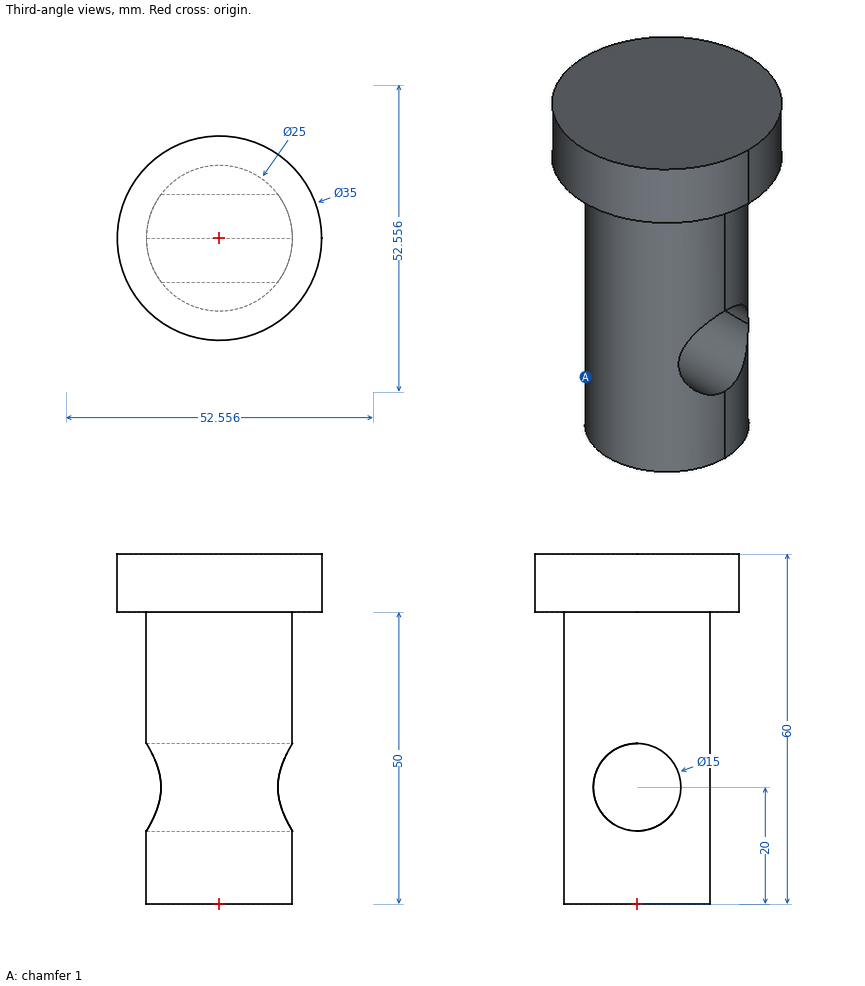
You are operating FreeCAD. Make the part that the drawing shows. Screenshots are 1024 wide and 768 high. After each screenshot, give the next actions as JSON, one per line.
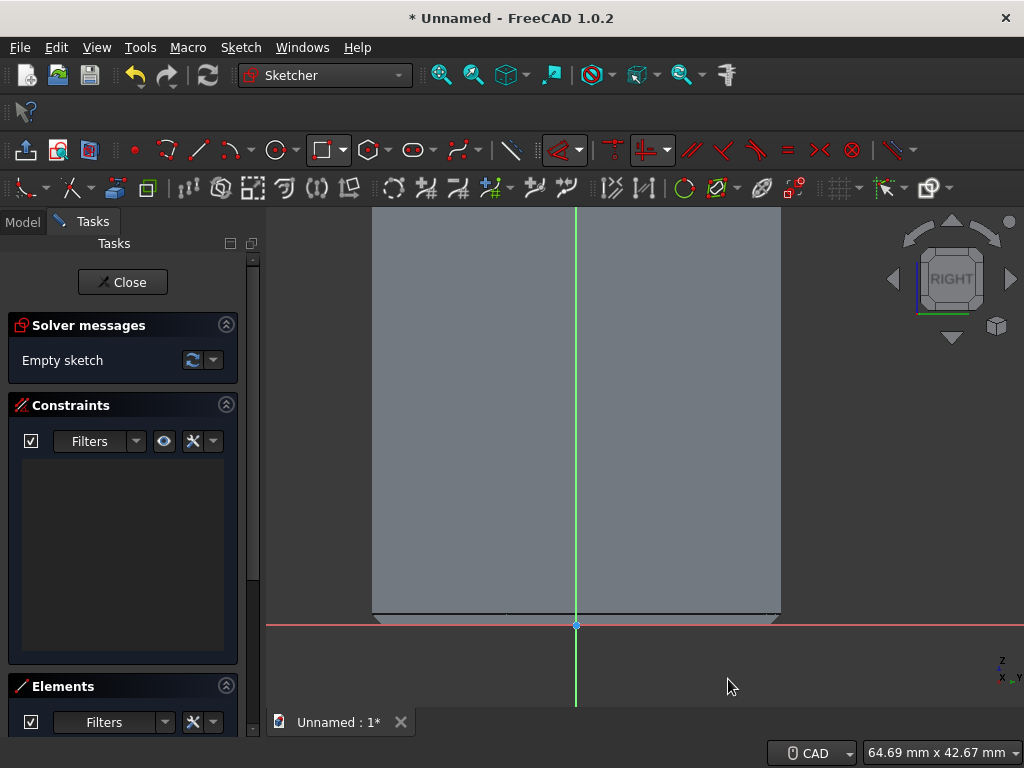
{"action": "left_click", "coordinate": [276, 150]}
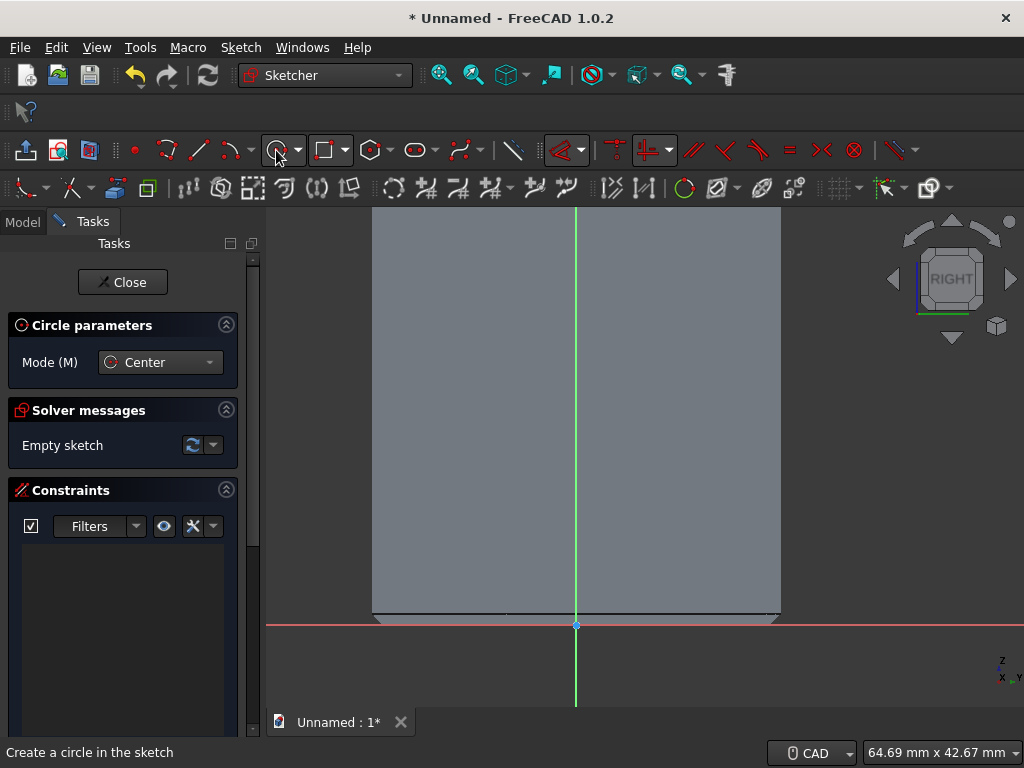
{"action": "left_click", "coordinate": [576, 391]}
{"action": "left_click", "coordinate": [638, 329]}
{"action": "key", "text": "Escape"}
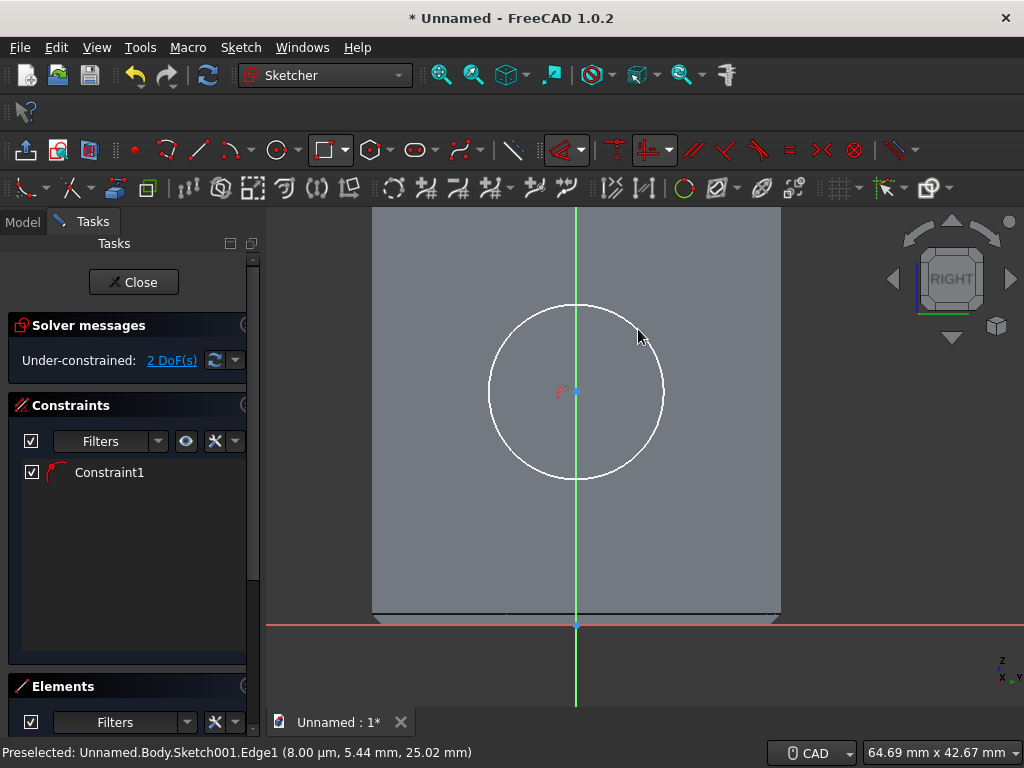
{"action": "left_click", "coordinate": [638, 330]}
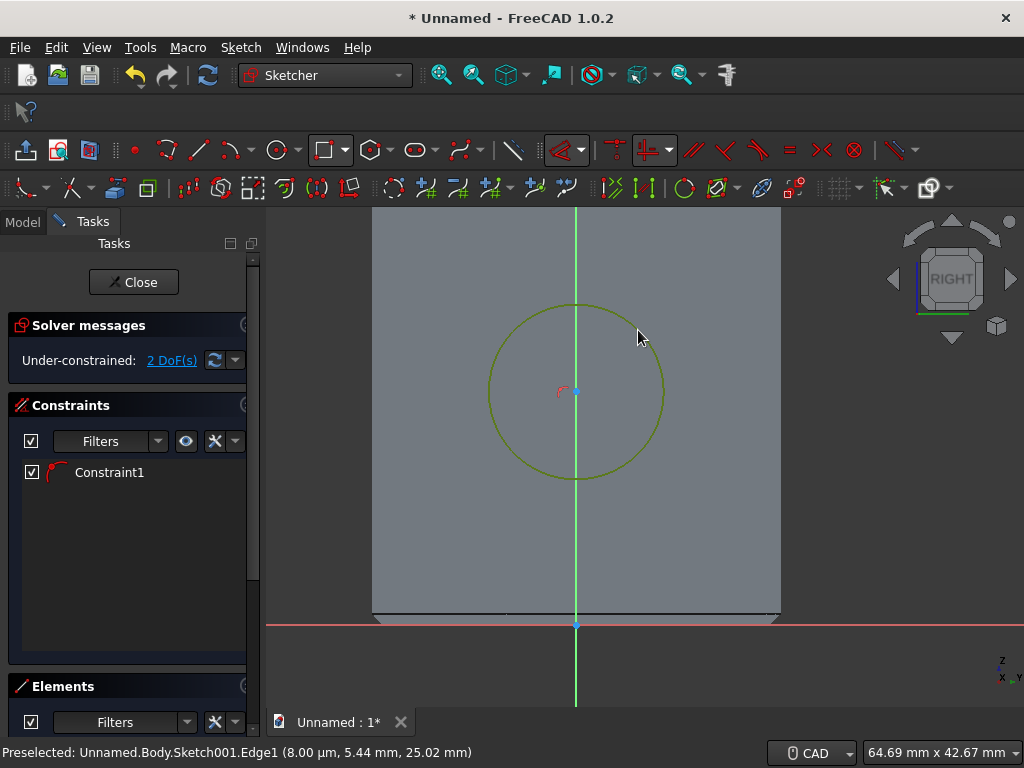
{"action": "key", "text": "k o"}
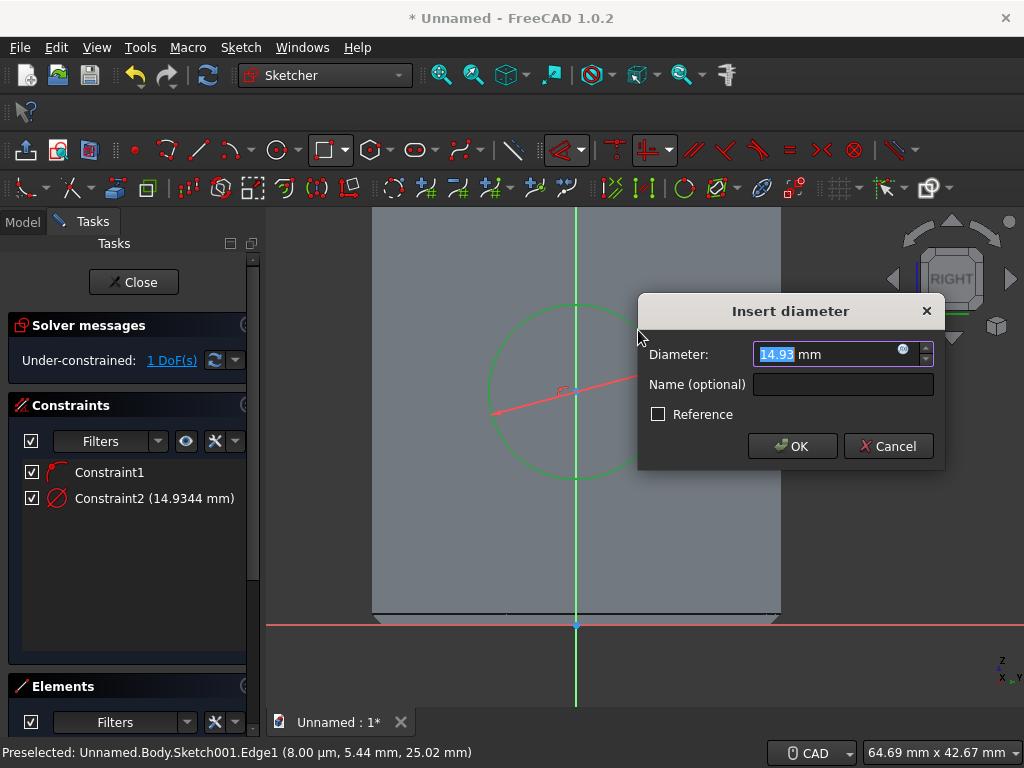
{"action": "type", "text": "15"}
{"action": "key", "text": "Return"}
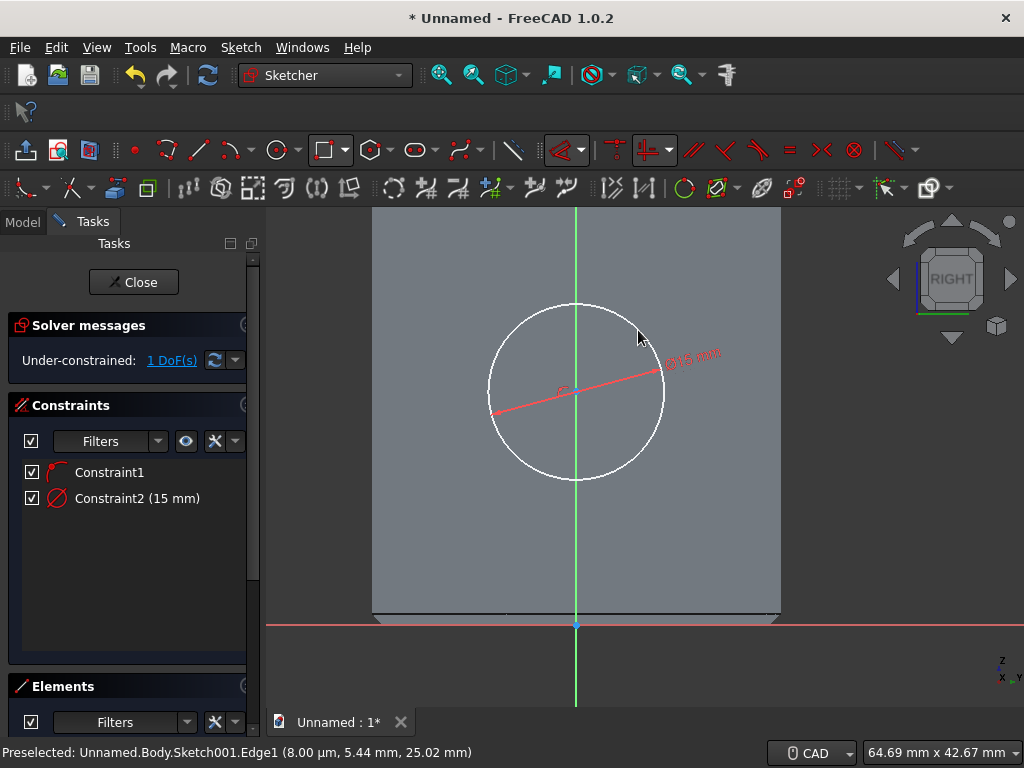
{"action": "left_click", "coordinate": [576, 392]}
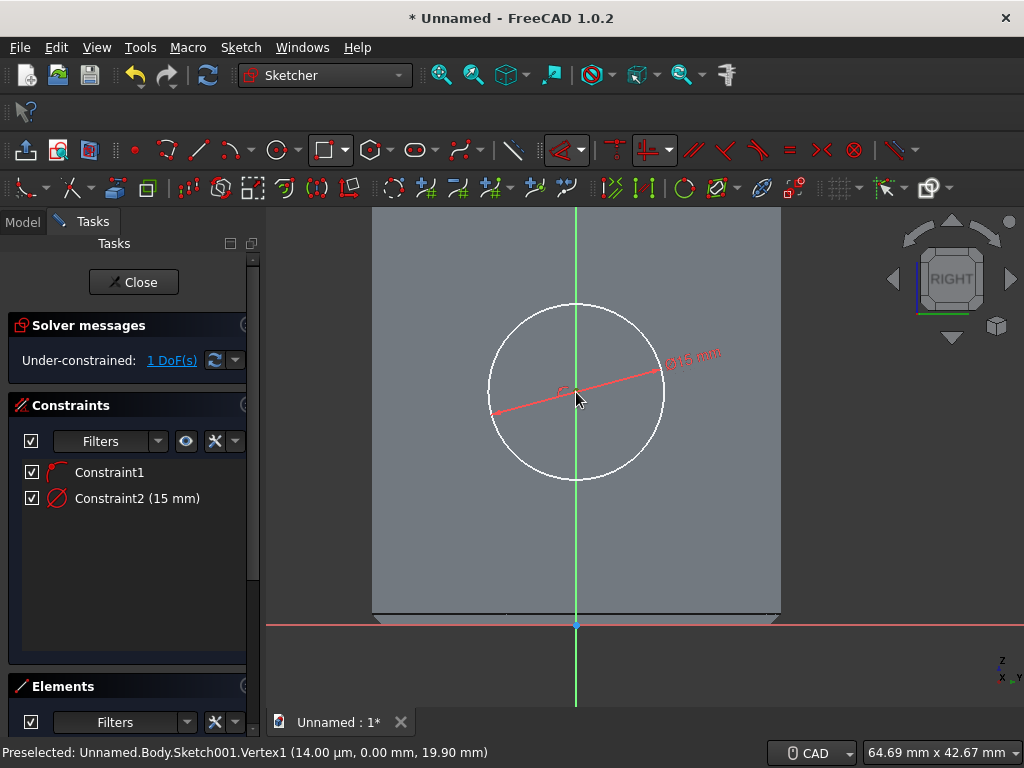
{"action": "left_click", "coordinate": [584, 150]}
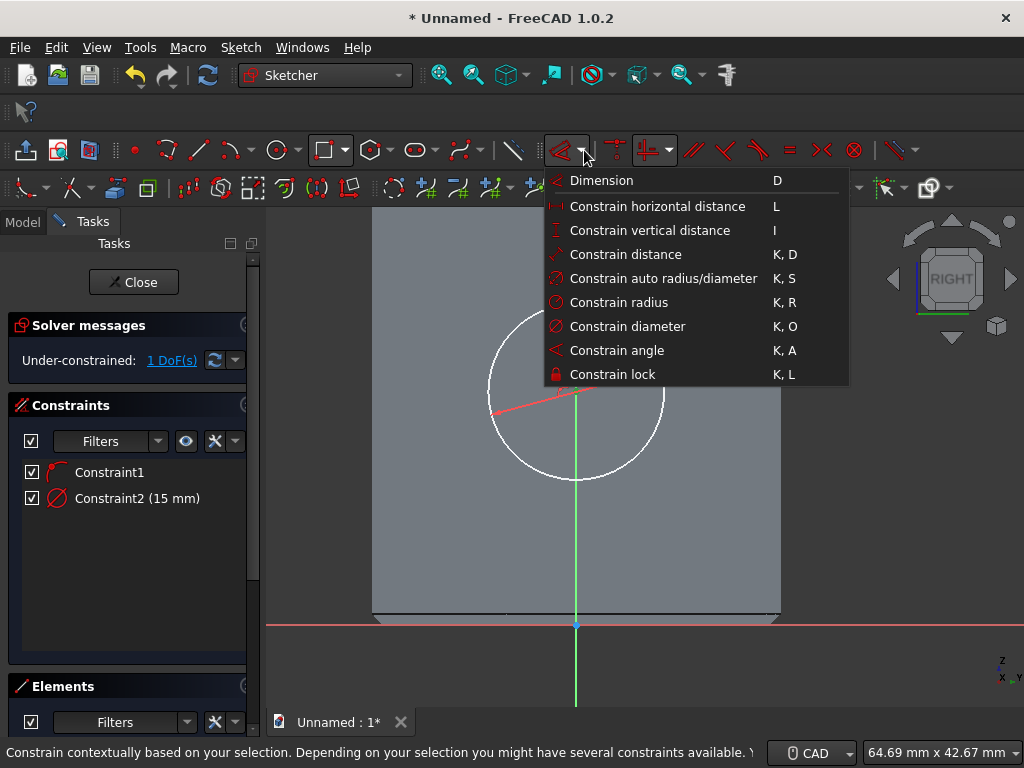
{"action": "left_click", "coordinate": [697, 230]}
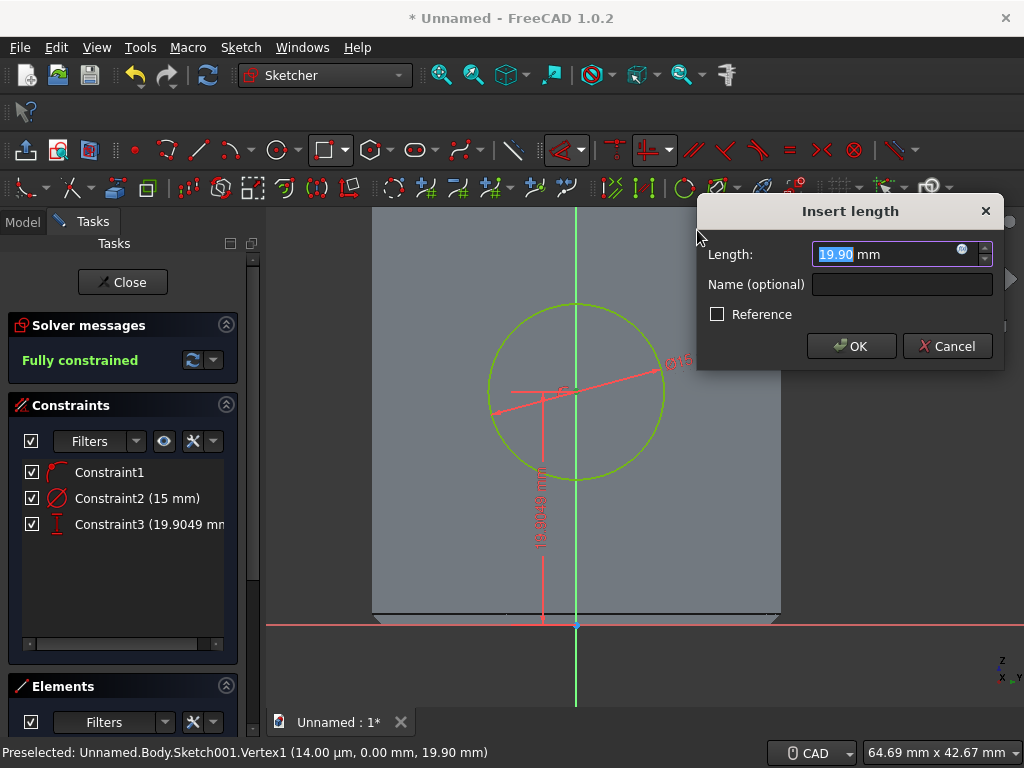
{"action": "type", "text": "20"}
{"action": "key", "text": "Return"}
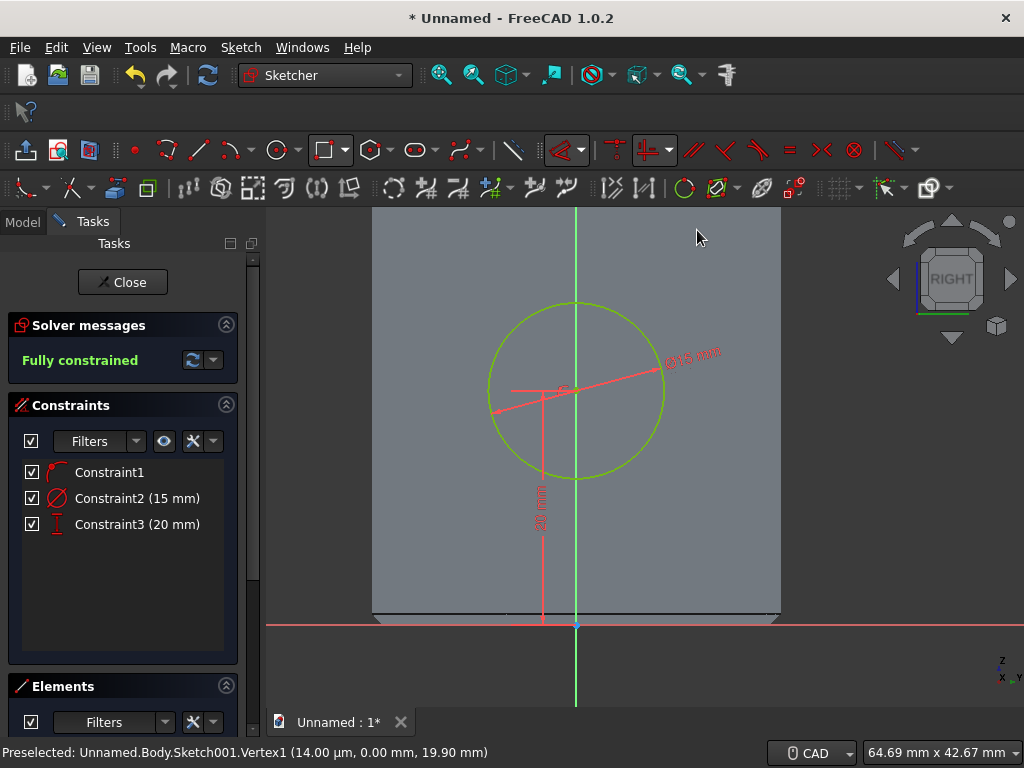
{"action": "left_click", "coordinate": [123, 282]}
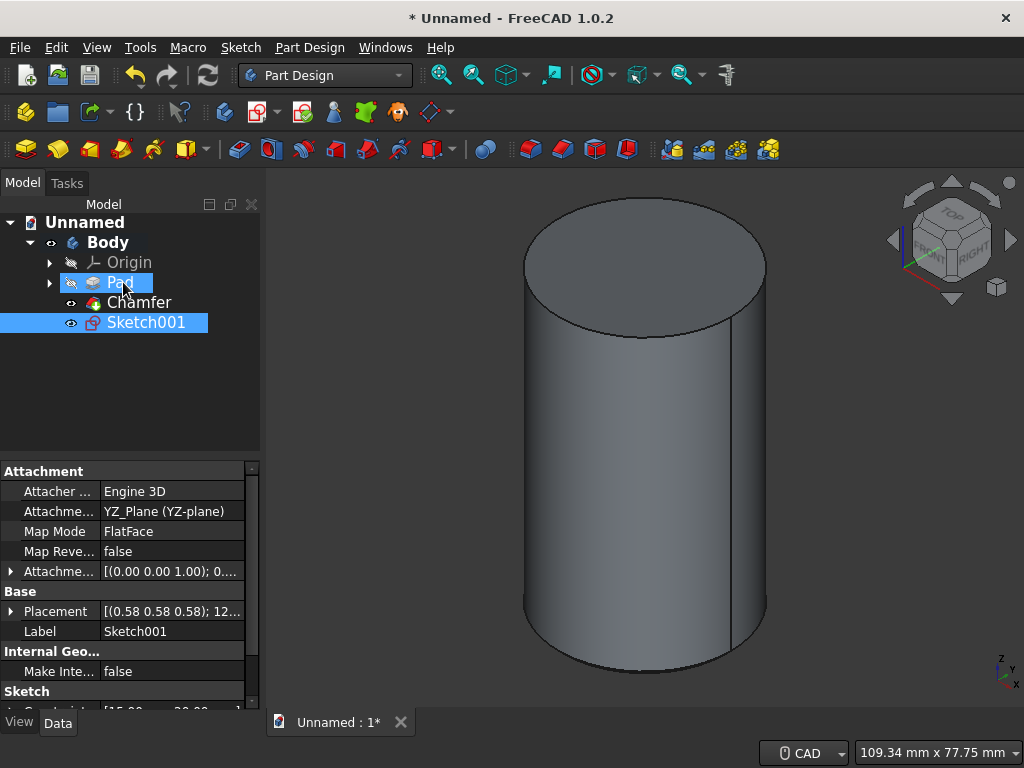
{"action": "left_click", "coordinate": [240, 150]}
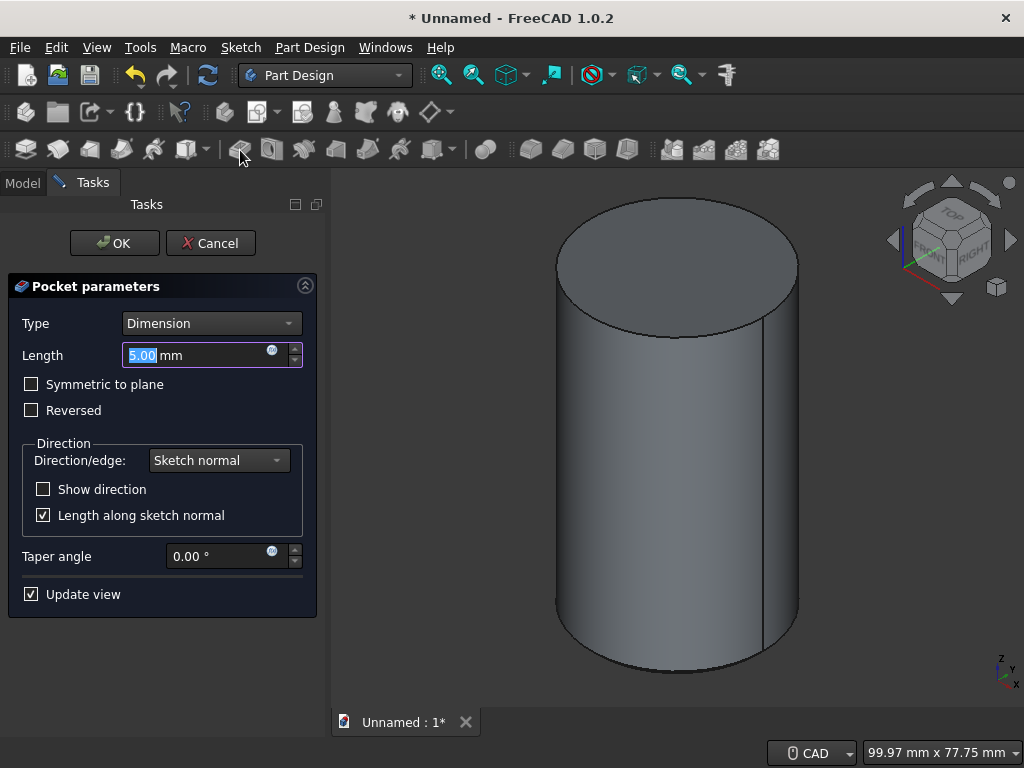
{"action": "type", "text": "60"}
{"action": "key", "text": "Tab"}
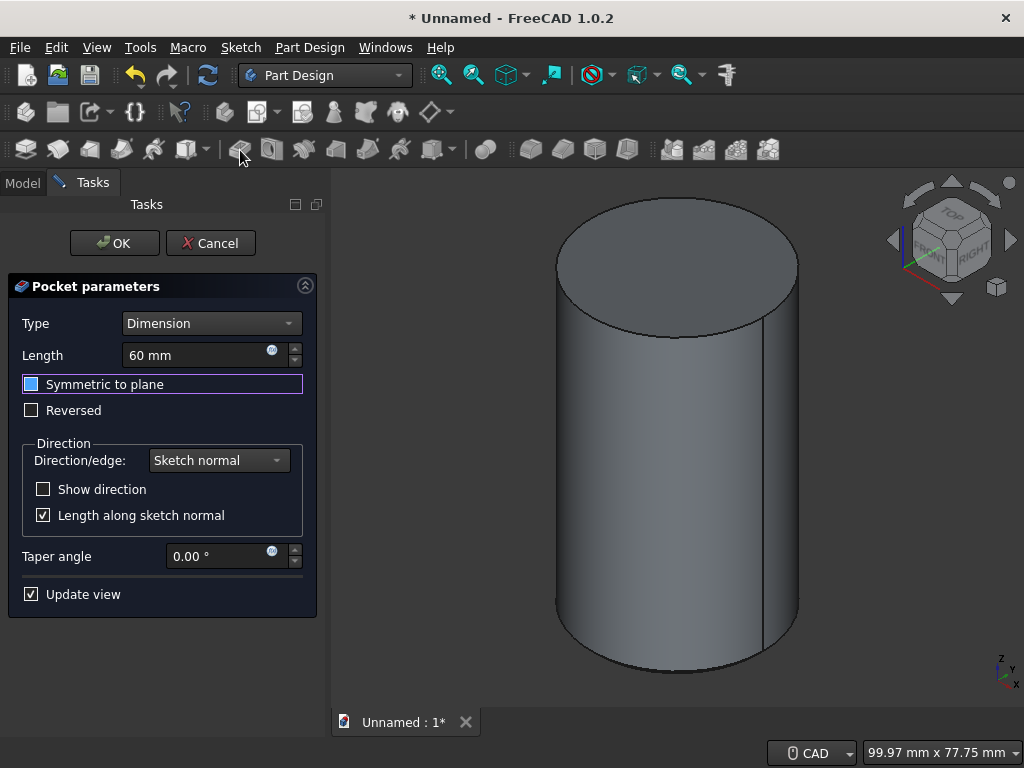
{"action": "left_click", "coordinate": [30, 384]}